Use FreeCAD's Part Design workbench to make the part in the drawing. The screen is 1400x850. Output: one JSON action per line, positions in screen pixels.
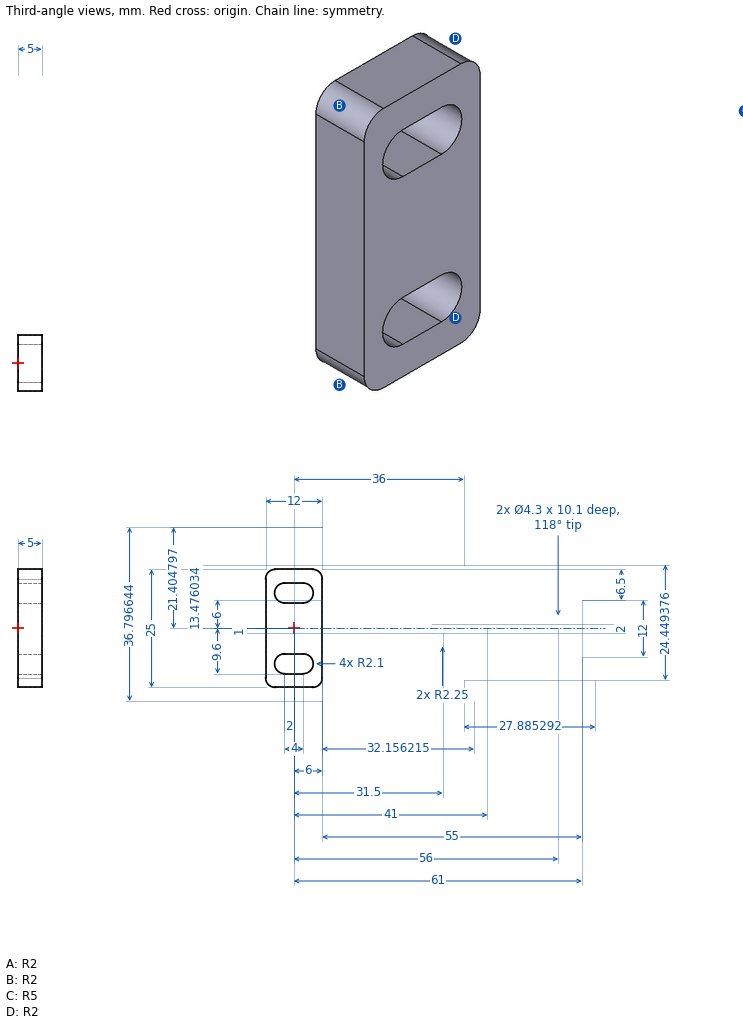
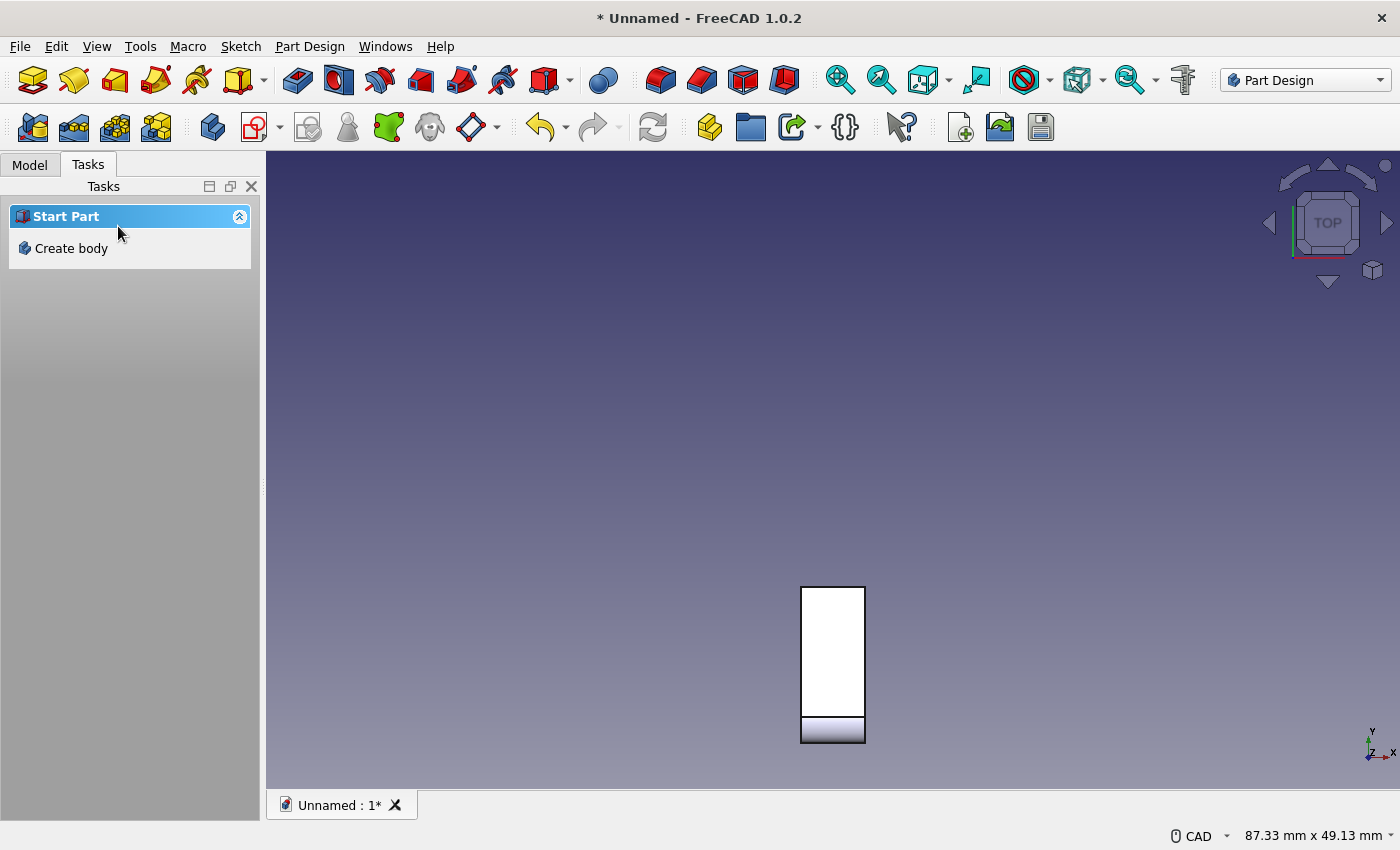
{"action": "key", "text": "v f"}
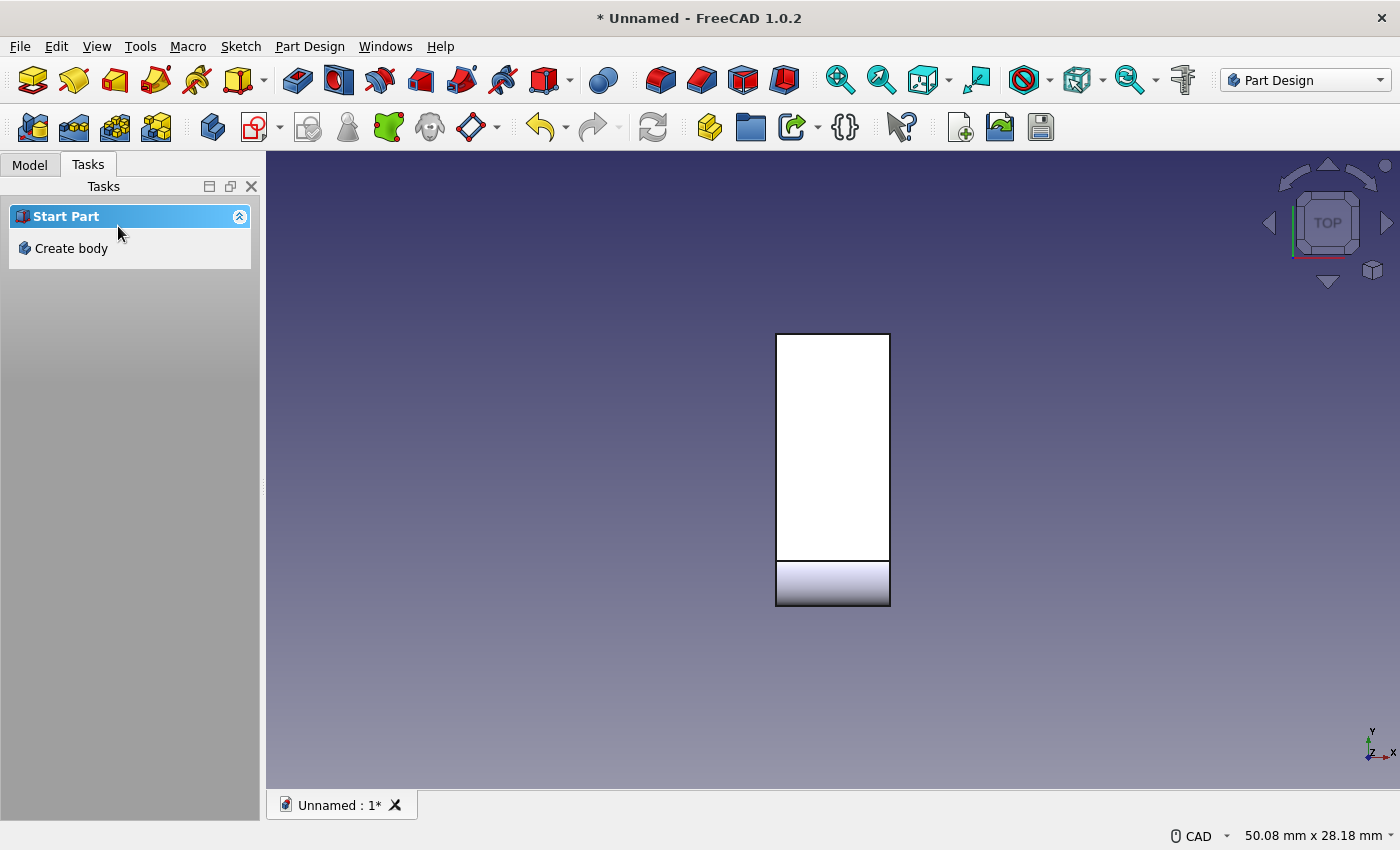
{"action": "left_click", "coordinate": [833, 333]}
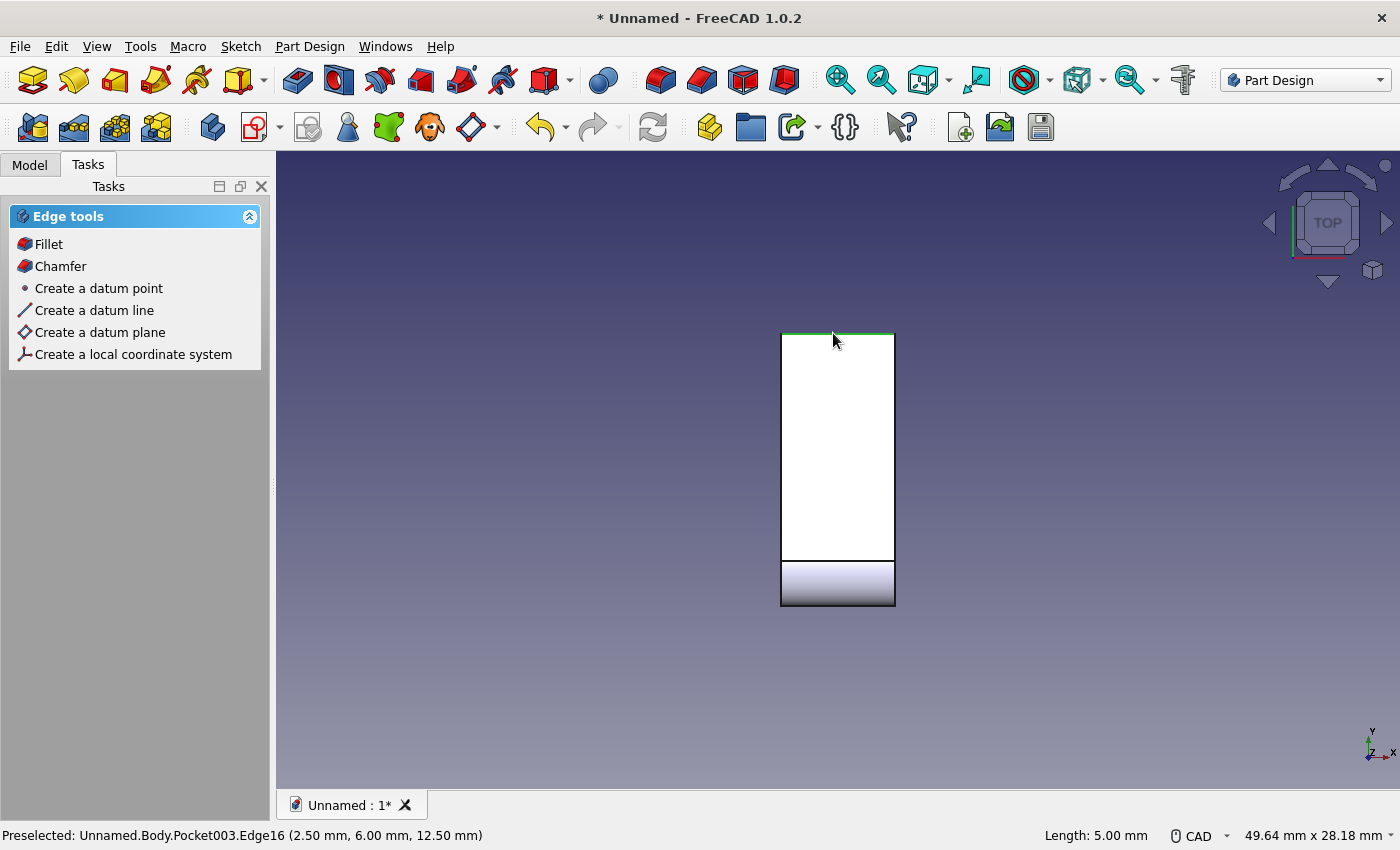
{"action": "key", "text": "0"}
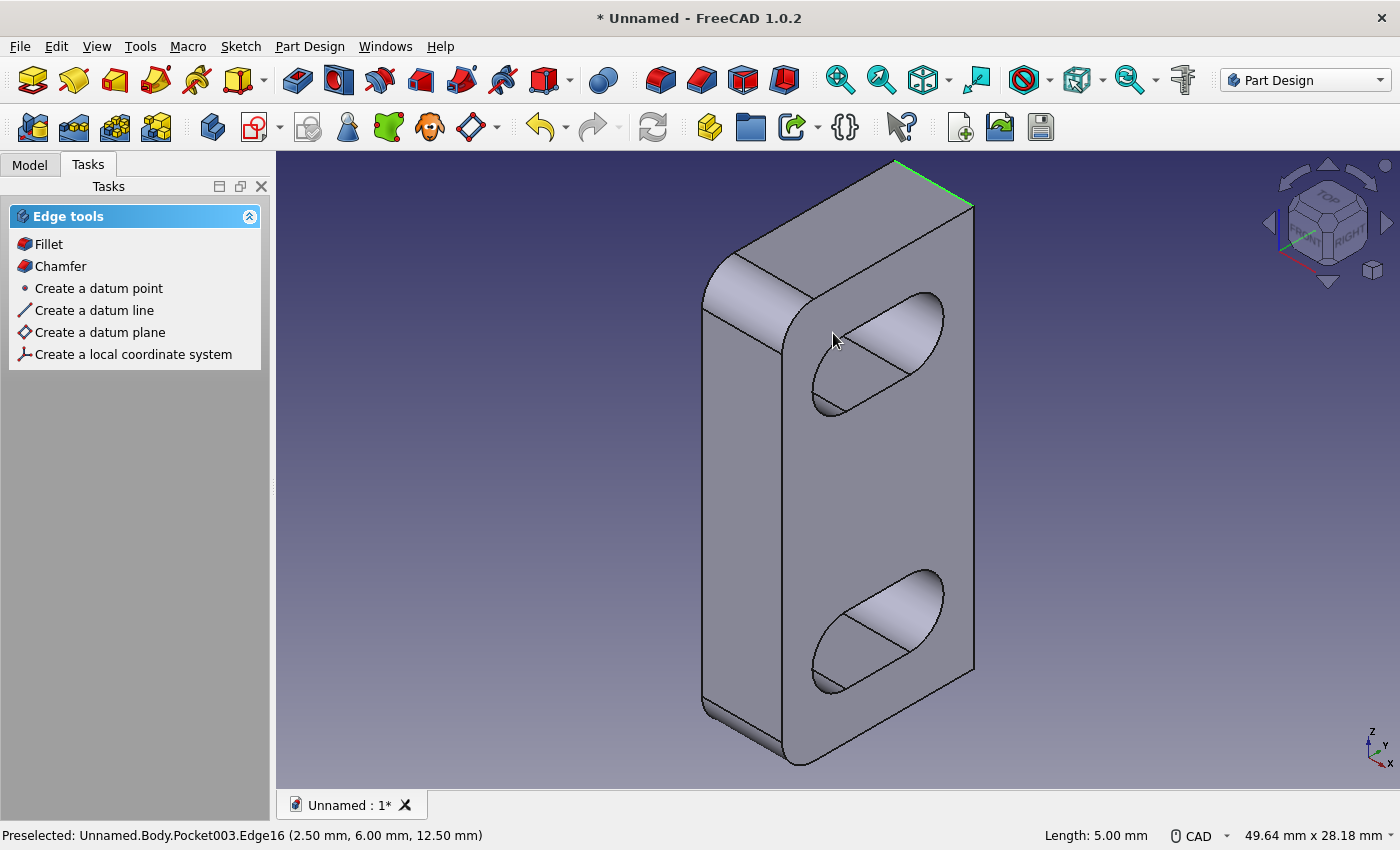
{"action": "key", "text": "1"}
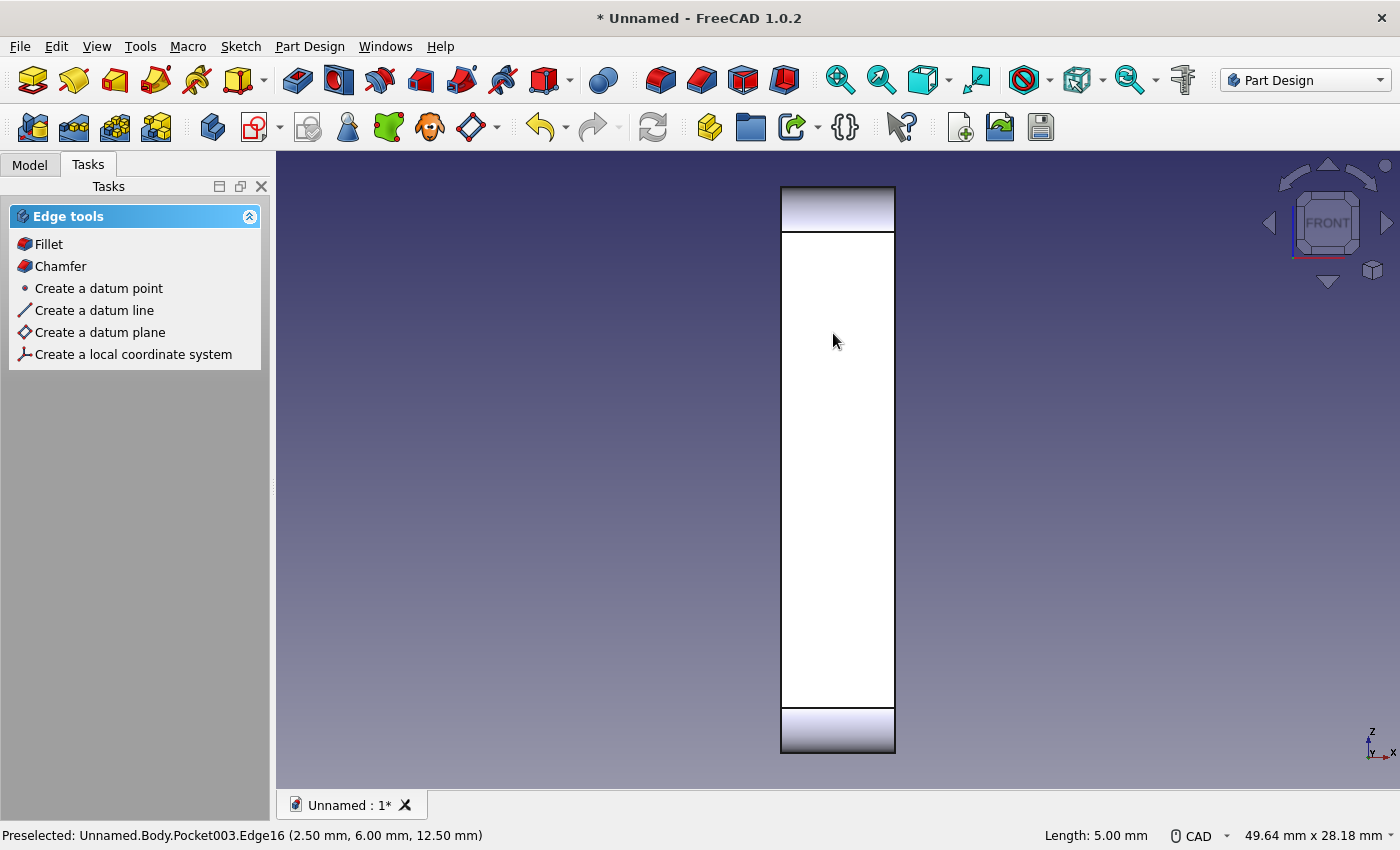
{"action": "key", "text": "3"}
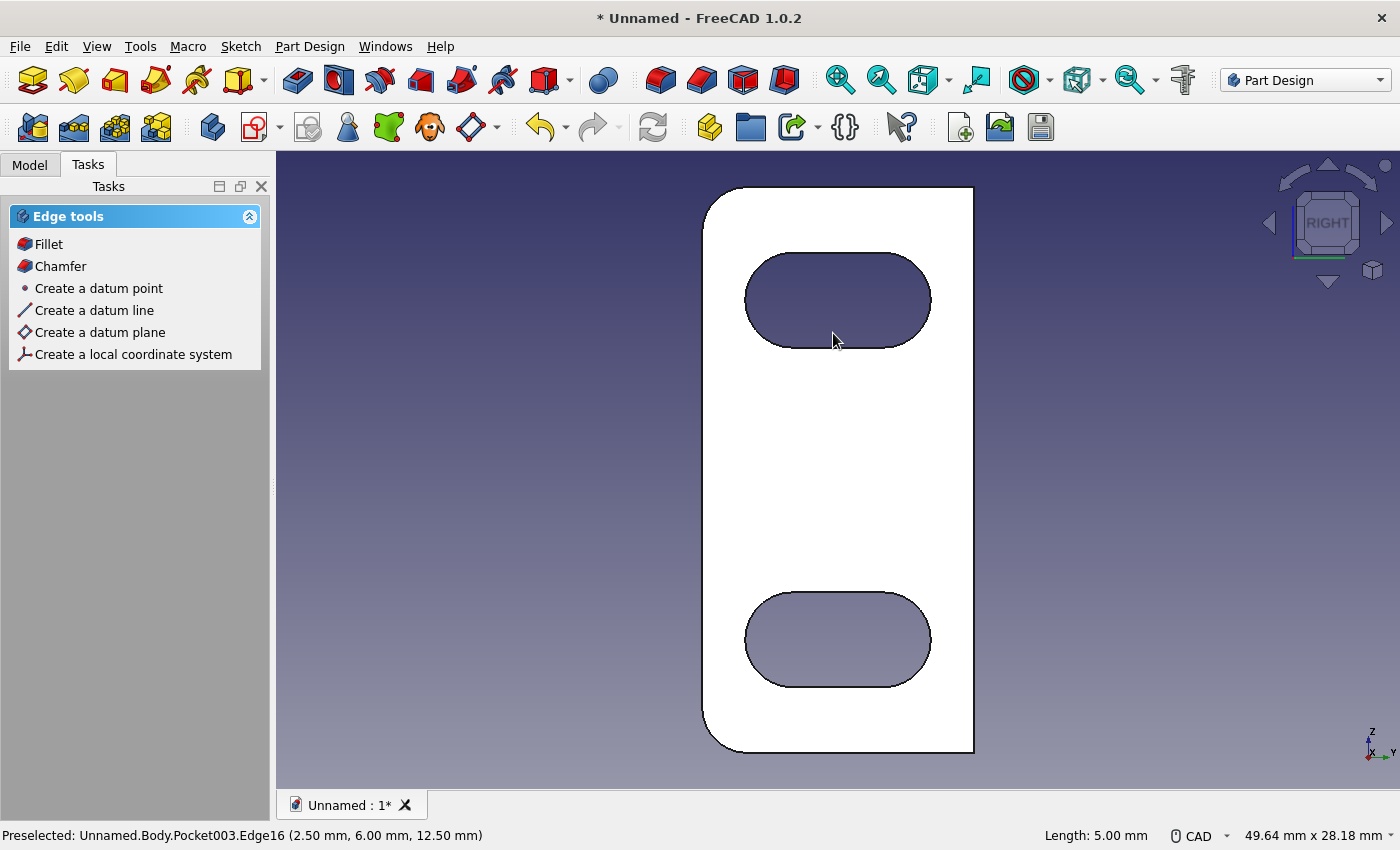
{"action": "key", "text": "5"}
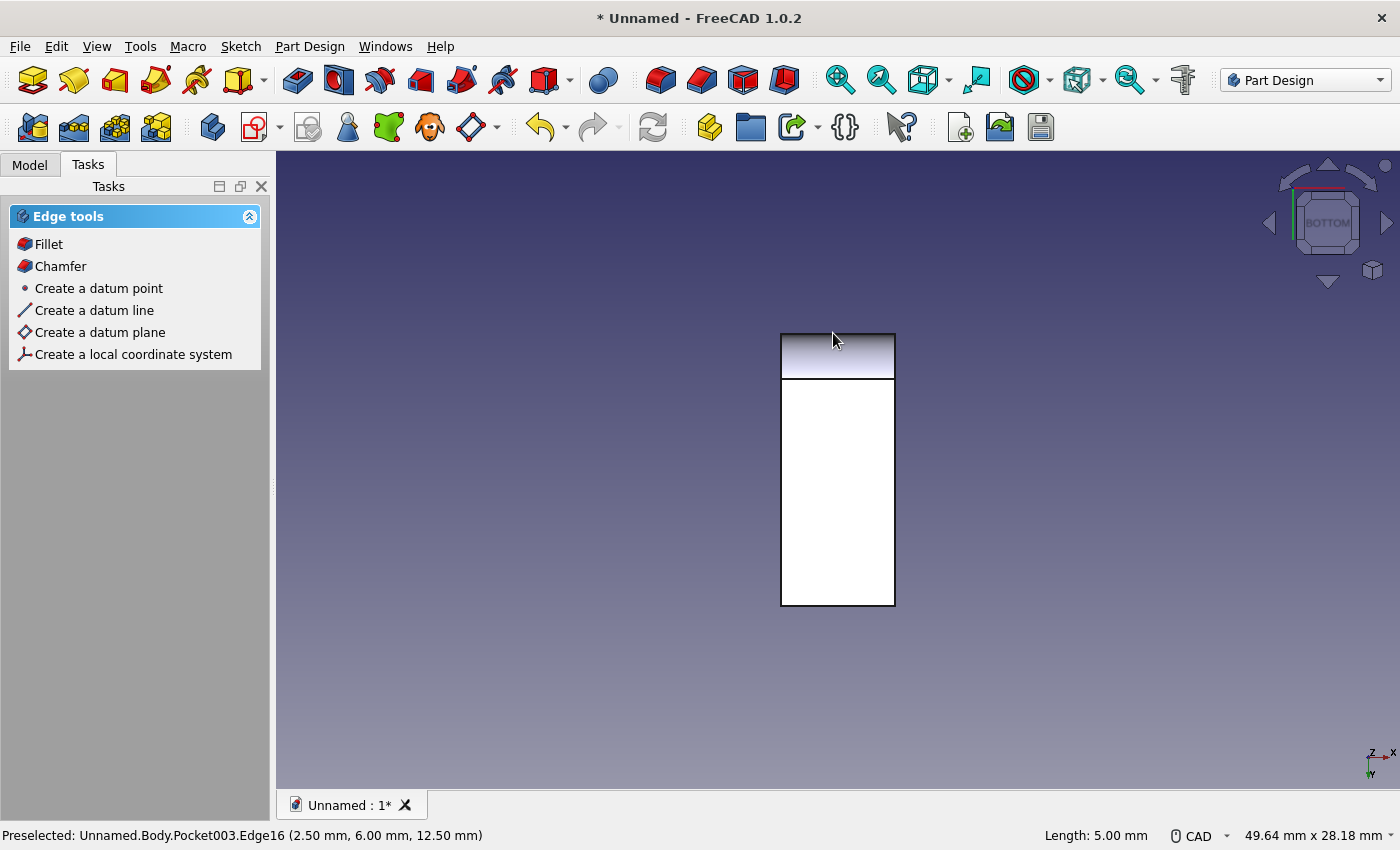
{"action": "left_click", "coordinate": [841, 80]}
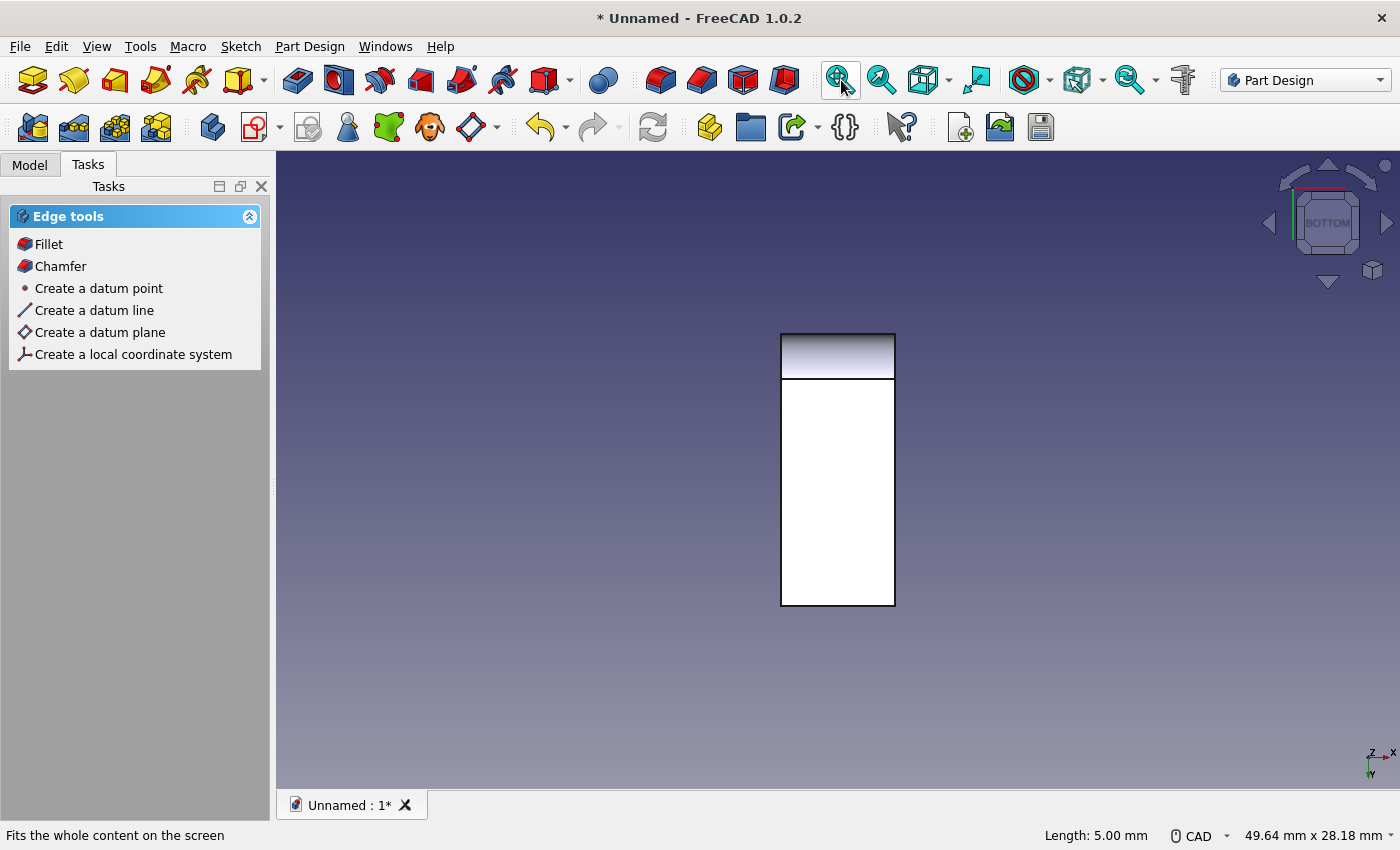
{"action": "left_click", "coordinate": [838, 605], "text": "ctrl"}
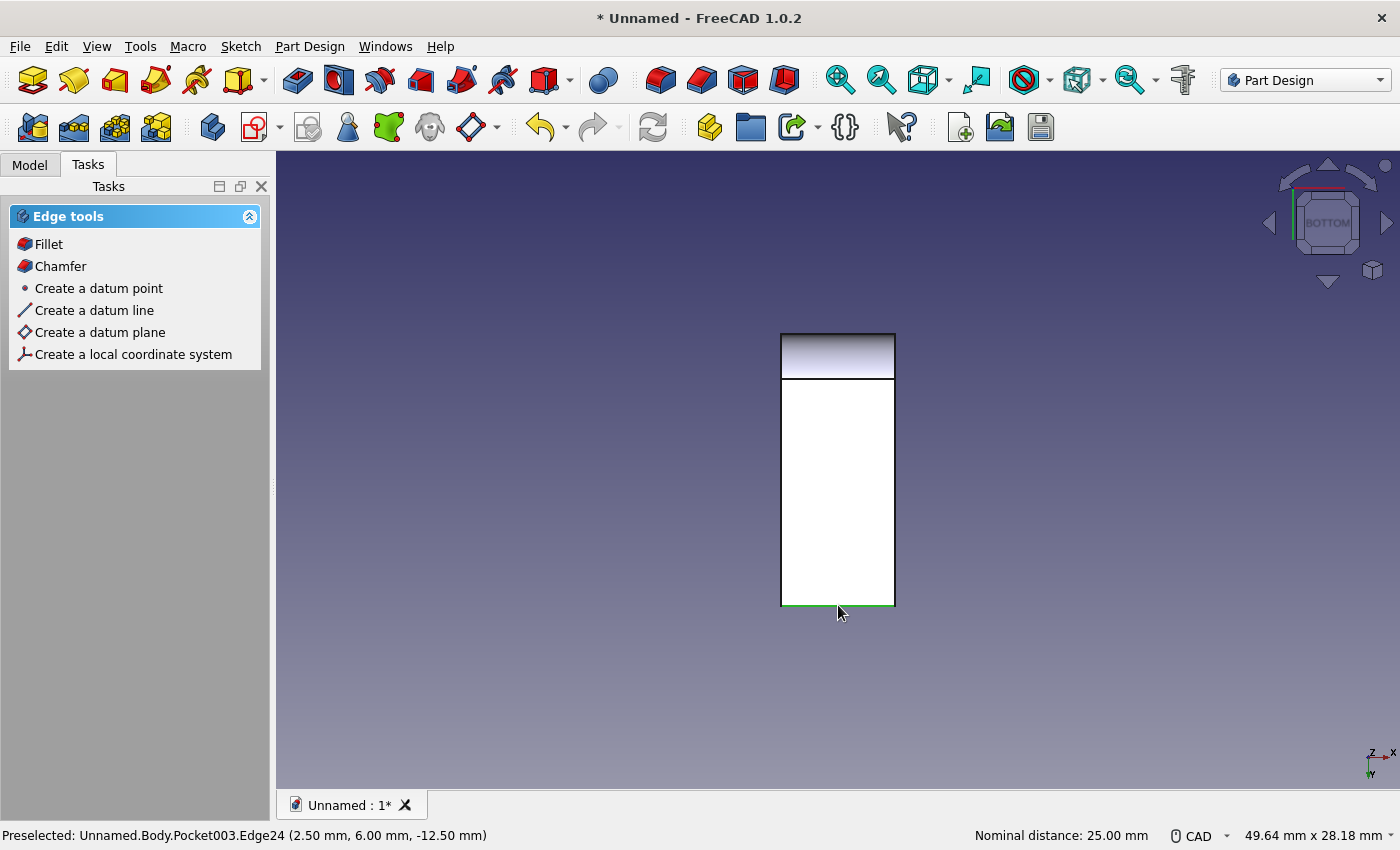
{"action": "left_click", "coordinate": [661, 80]}